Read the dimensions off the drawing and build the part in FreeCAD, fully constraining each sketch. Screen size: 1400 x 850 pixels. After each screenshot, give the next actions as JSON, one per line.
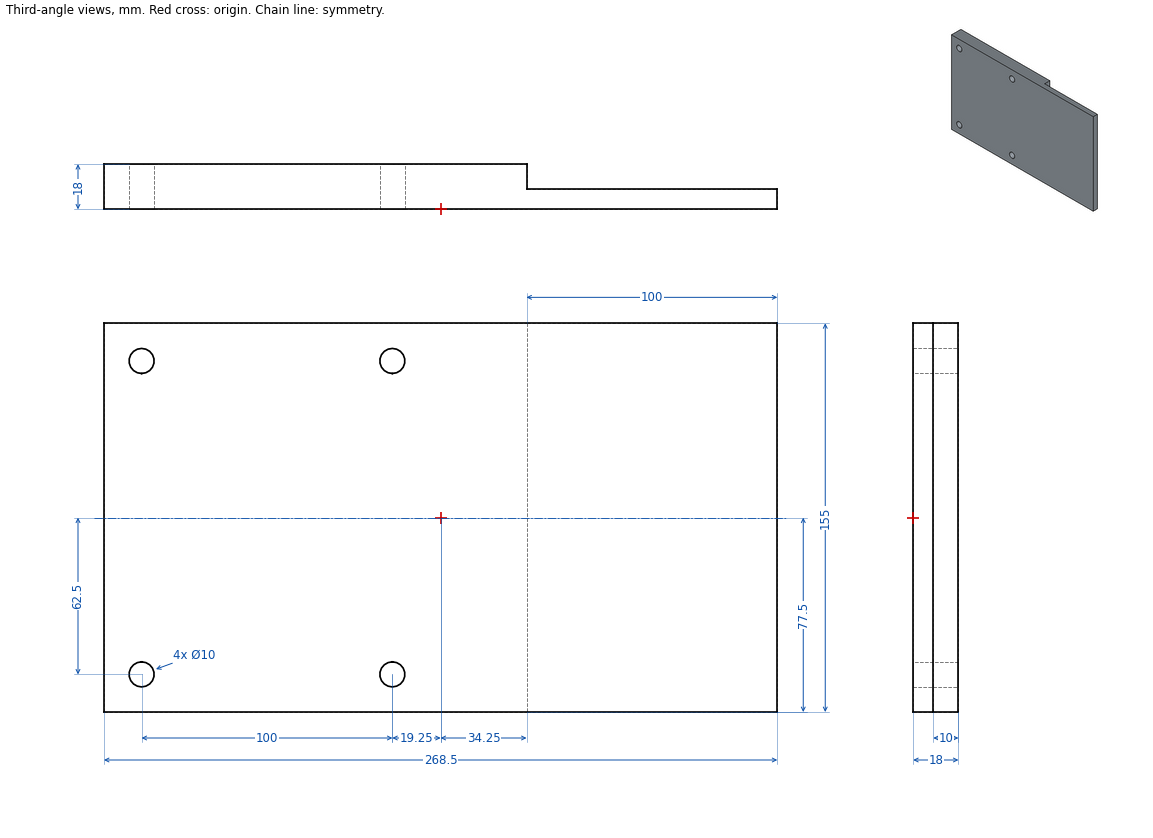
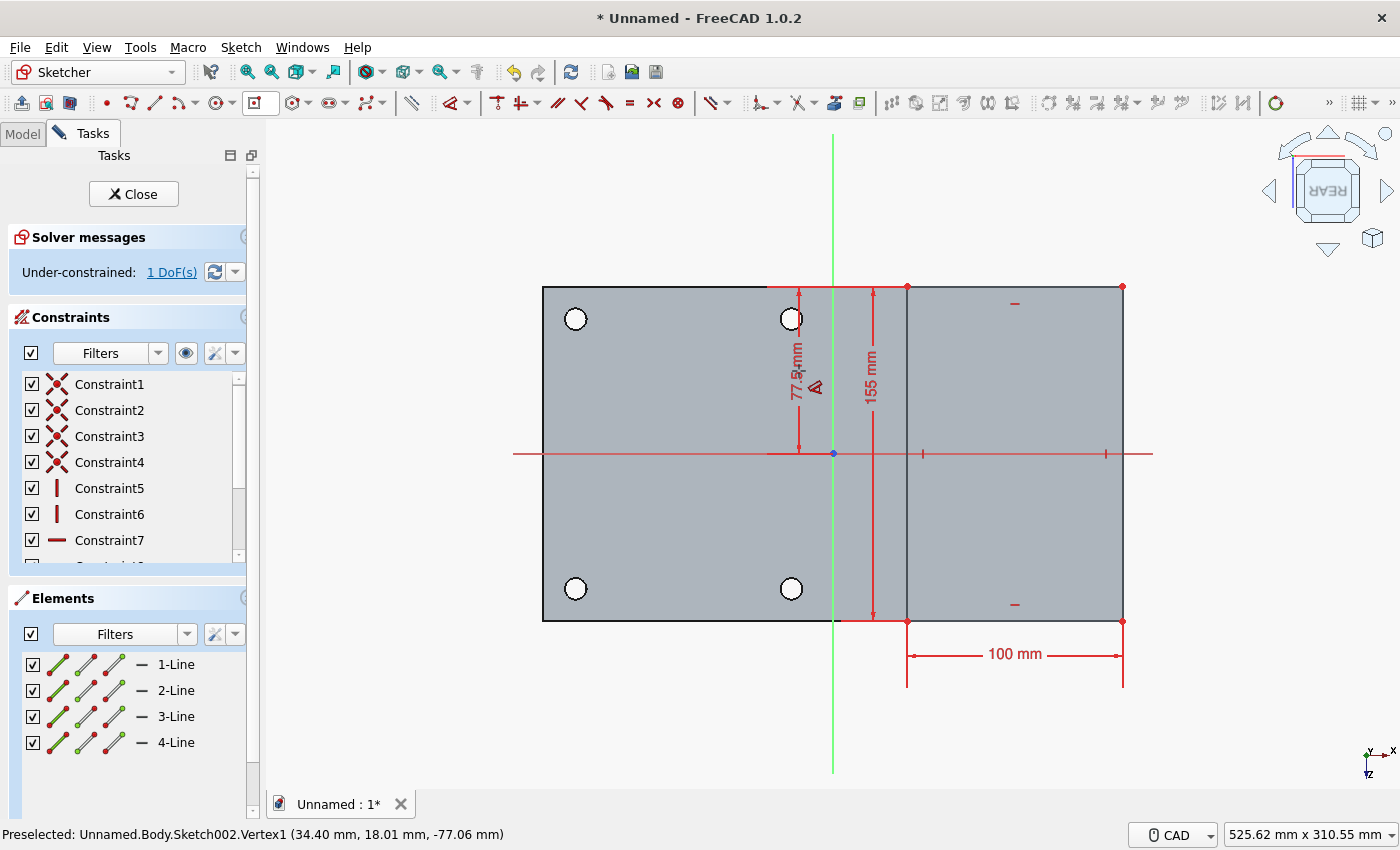
{"action": "left_click", "coordinate": [907, 287]}
{"action": "left_click", "coordinate": [870, 253]}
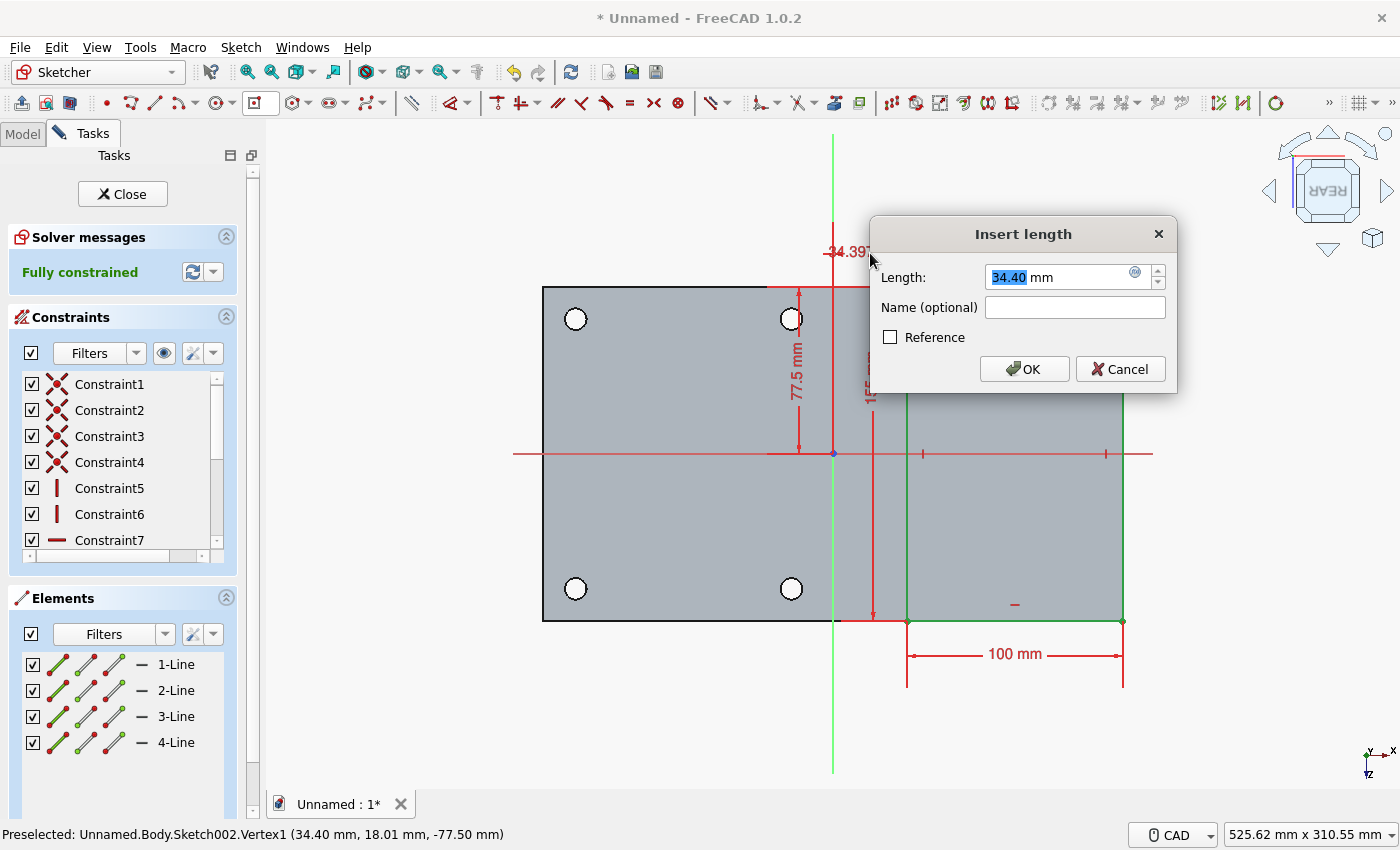
{"action": "type", "text": "34.25"}
{"action": "key", "text": "Return"}
{"action": "key", "text": "Escape"}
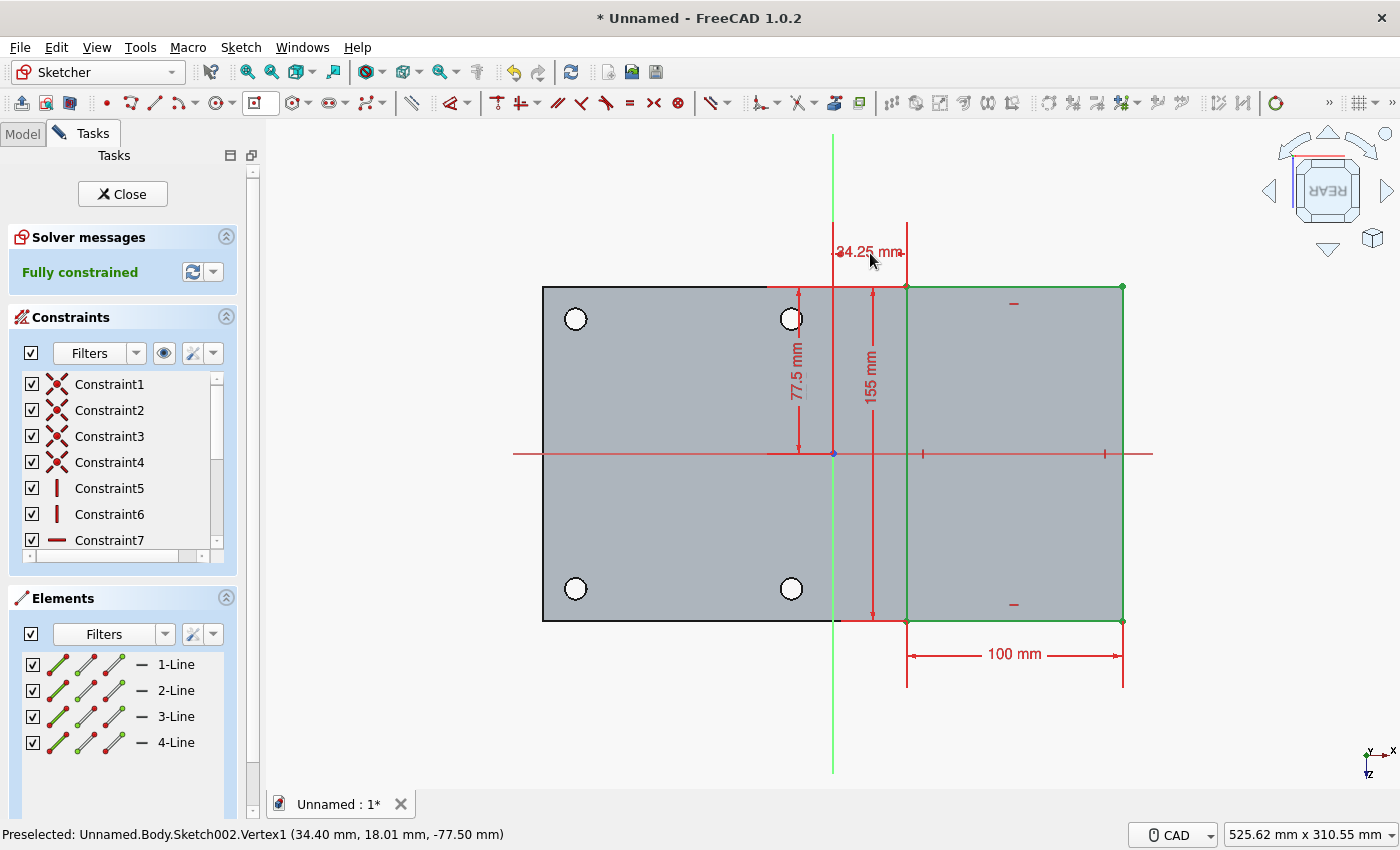
{"action": "left_click", "coordinate": [123, 194]}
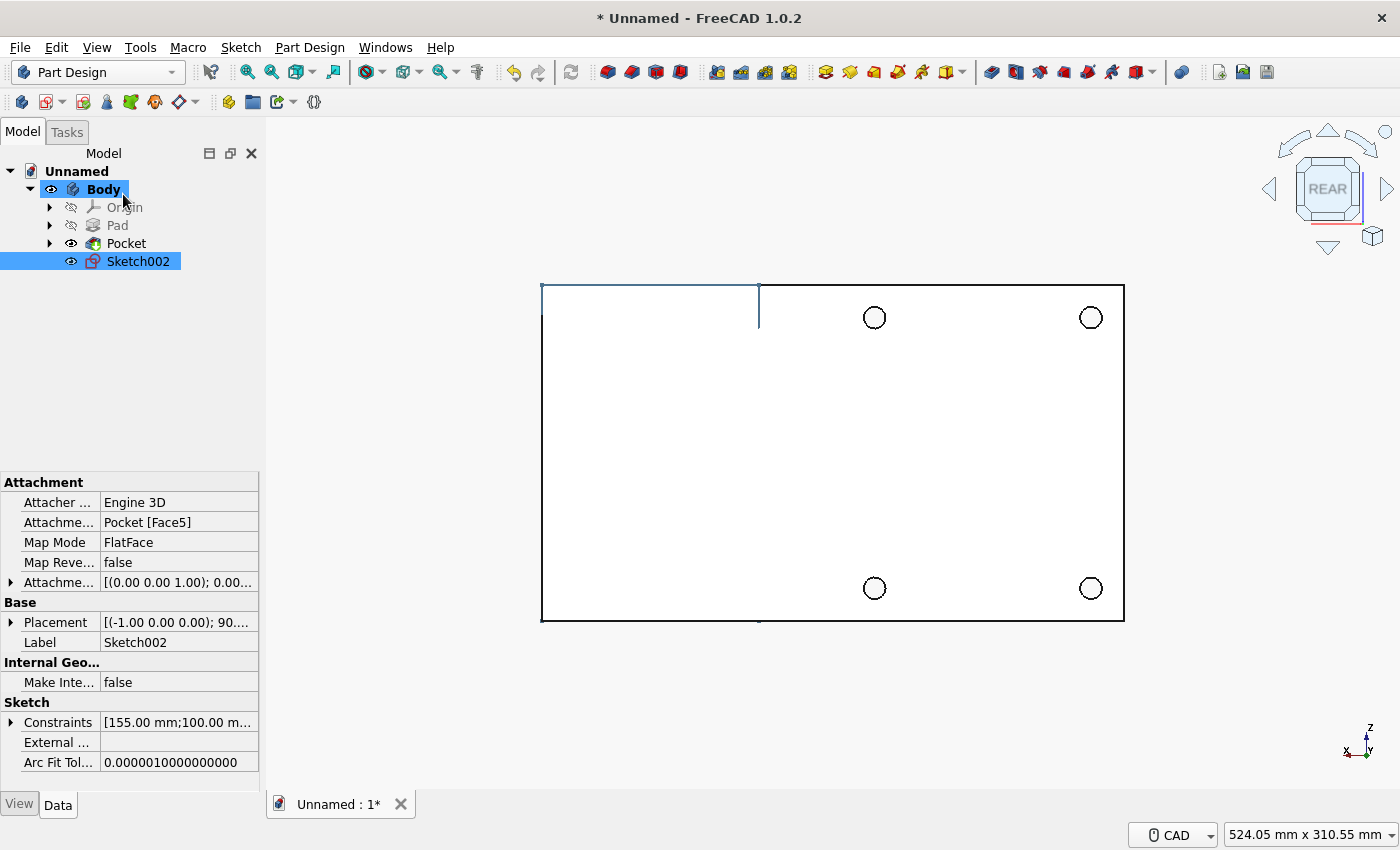
{"action": "left_click", "coordinate": [992, 72]}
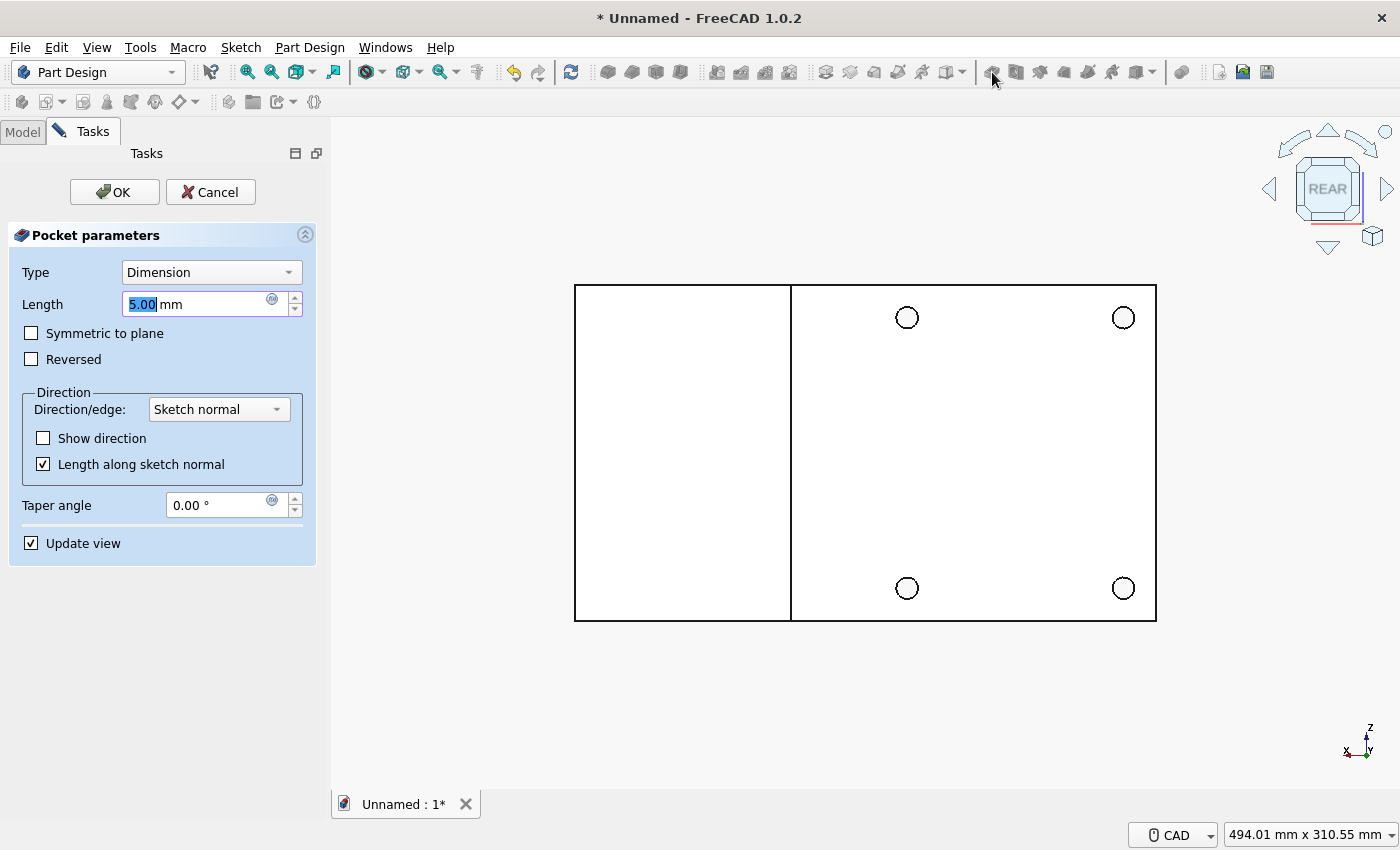
{"action": "type", "text": "10"}
{"action": "key", "text": "Tab"}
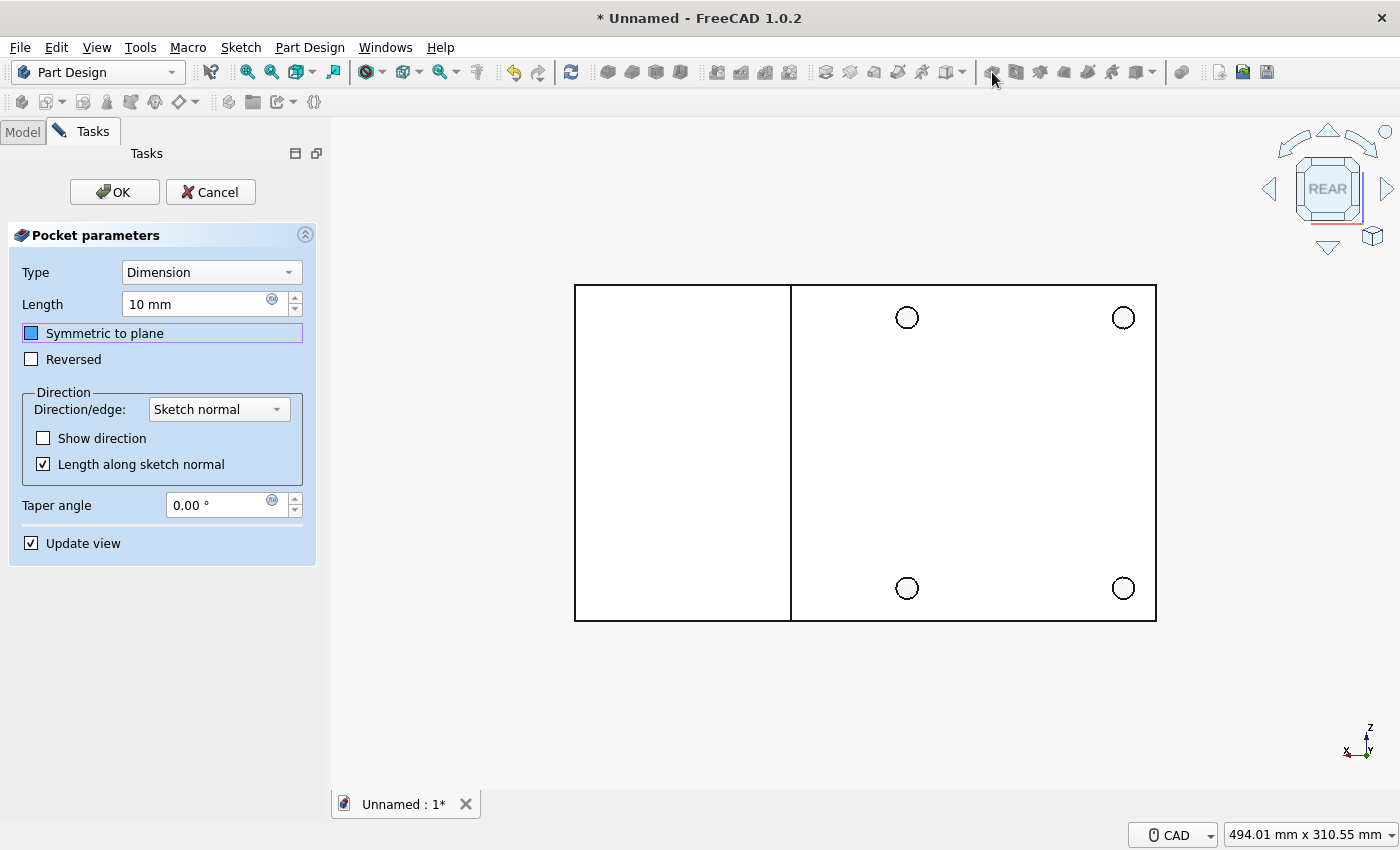
{"action": "left_click", "coordinate": [115, 192]}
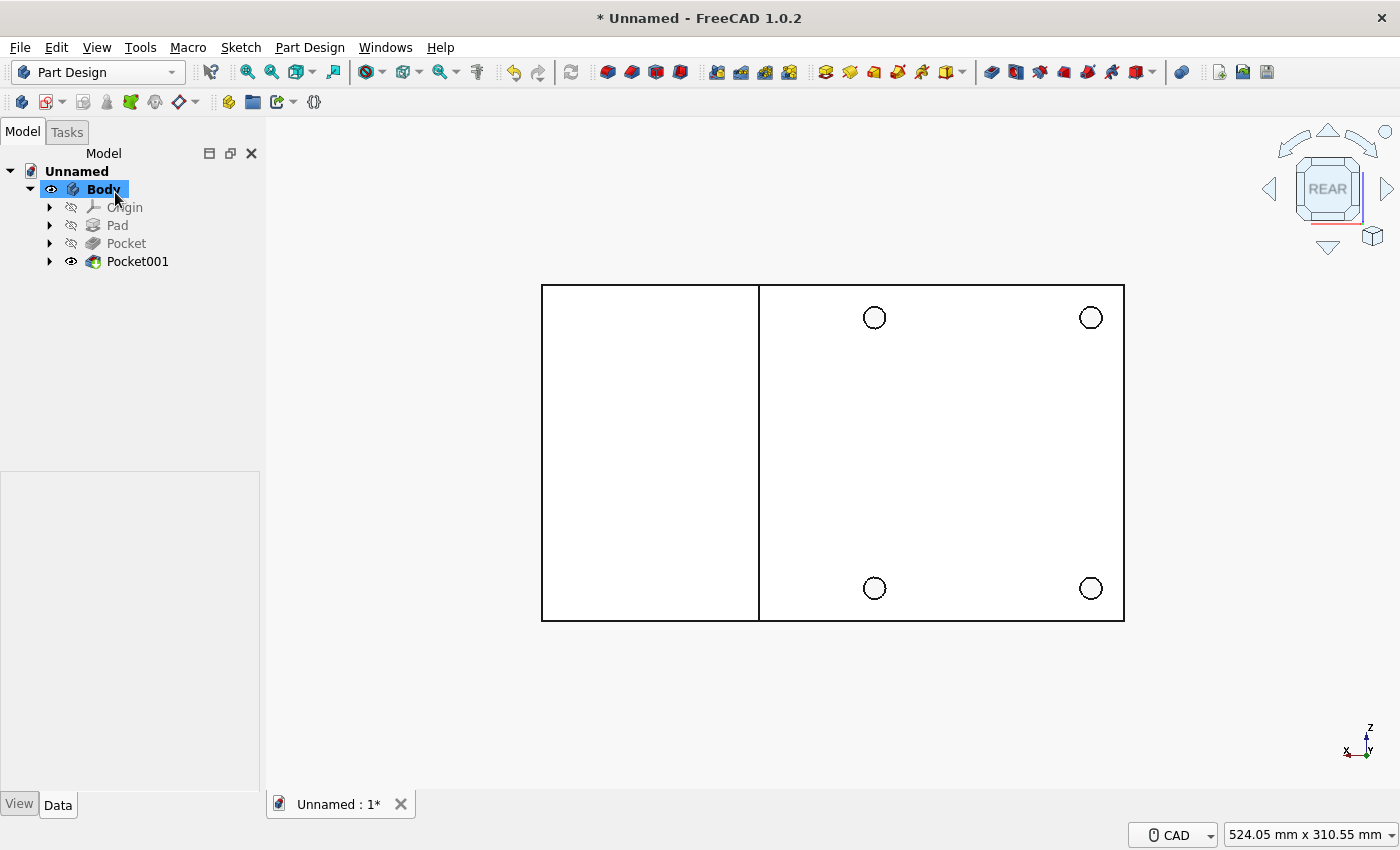
{"action": "key", "text": "0"}